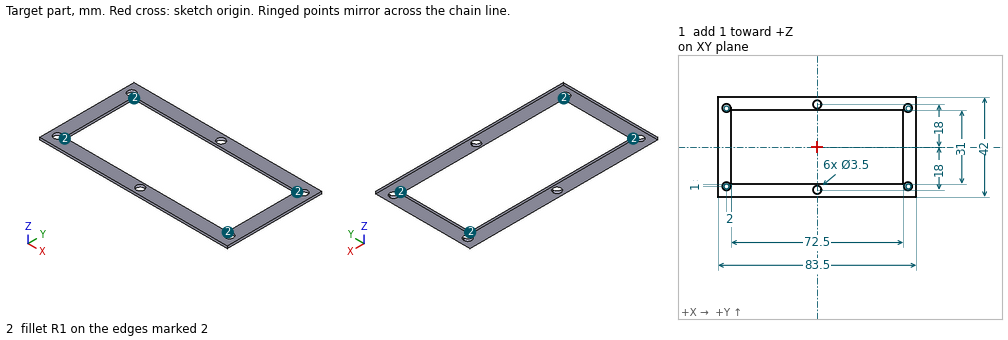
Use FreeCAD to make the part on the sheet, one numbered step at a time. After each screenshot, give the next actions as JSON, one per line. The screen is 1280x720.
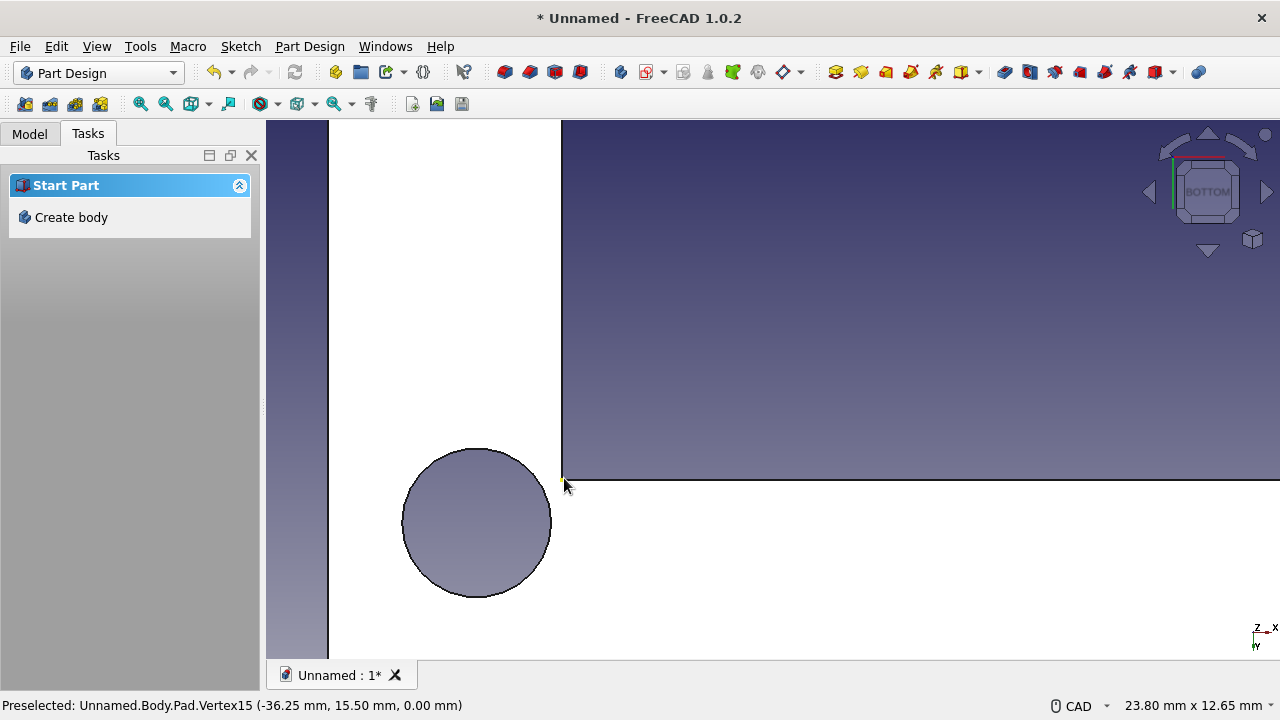
{"action": "left_click", "coordinate": [141, 104]}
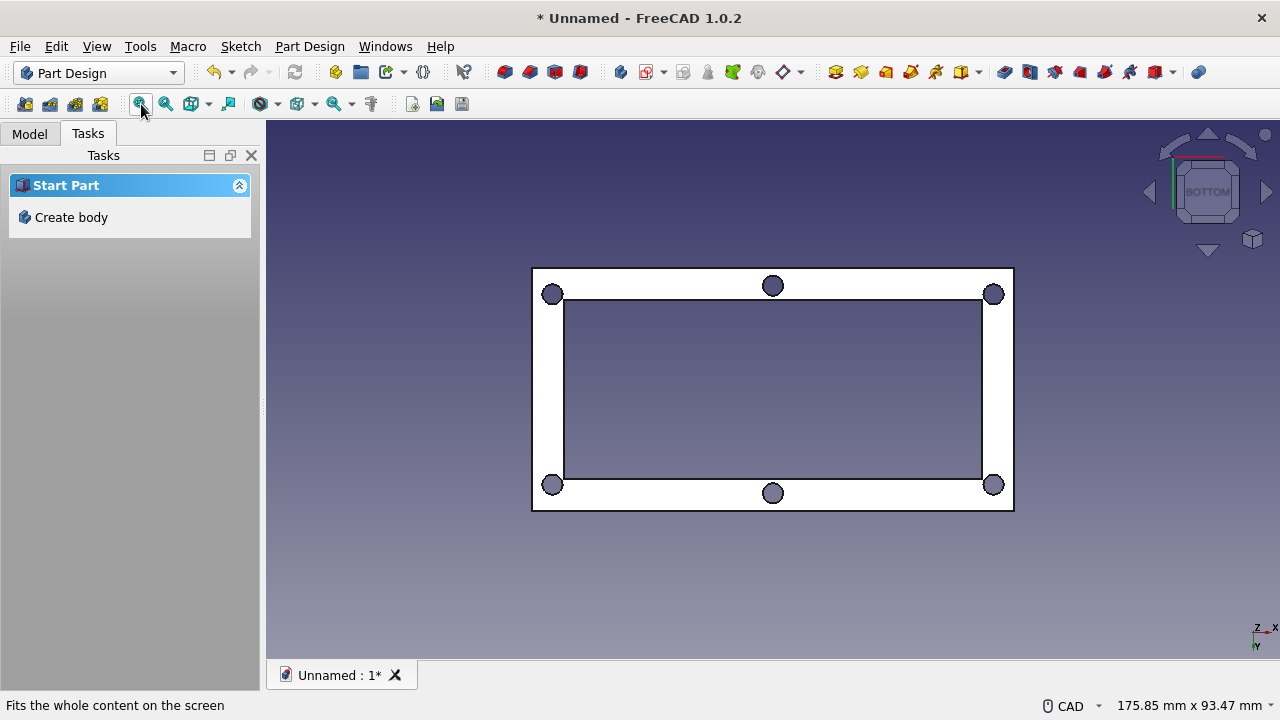
{"action": "key", "text": "4"}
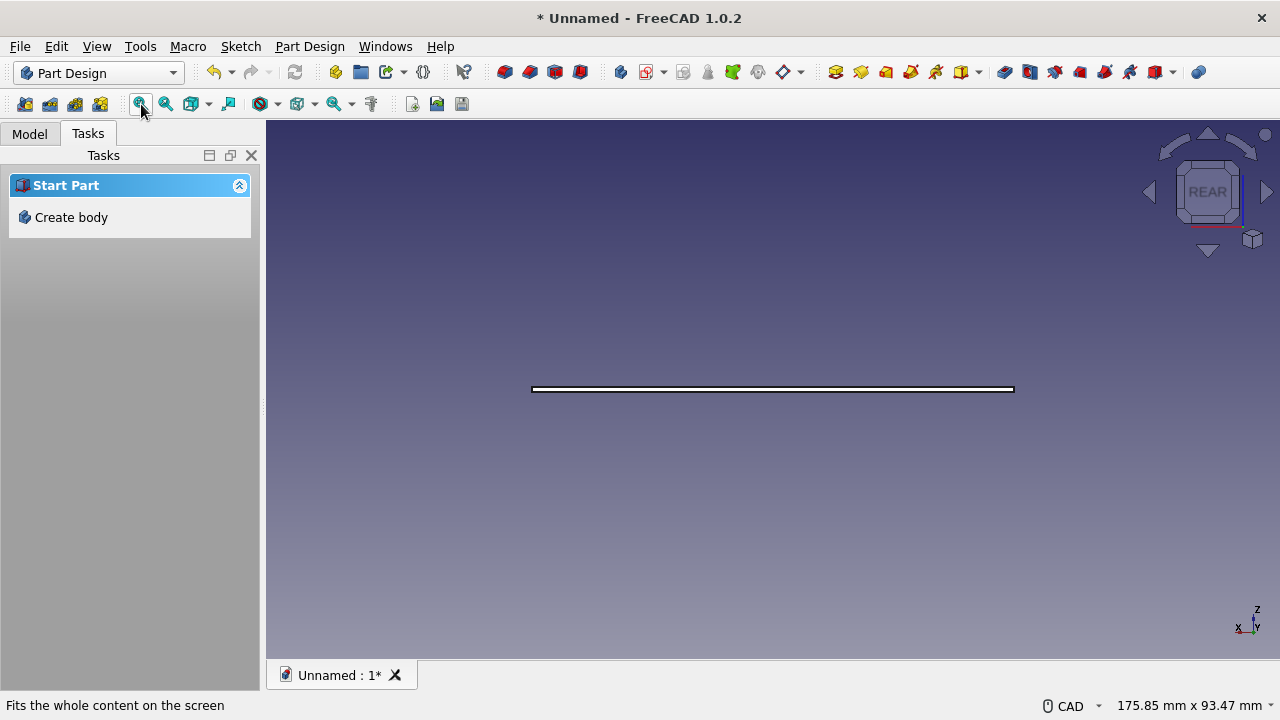
{"action": "scroll", "coordinate": [982, 389], "scroll_direction": "up", "scroll_amount": 10}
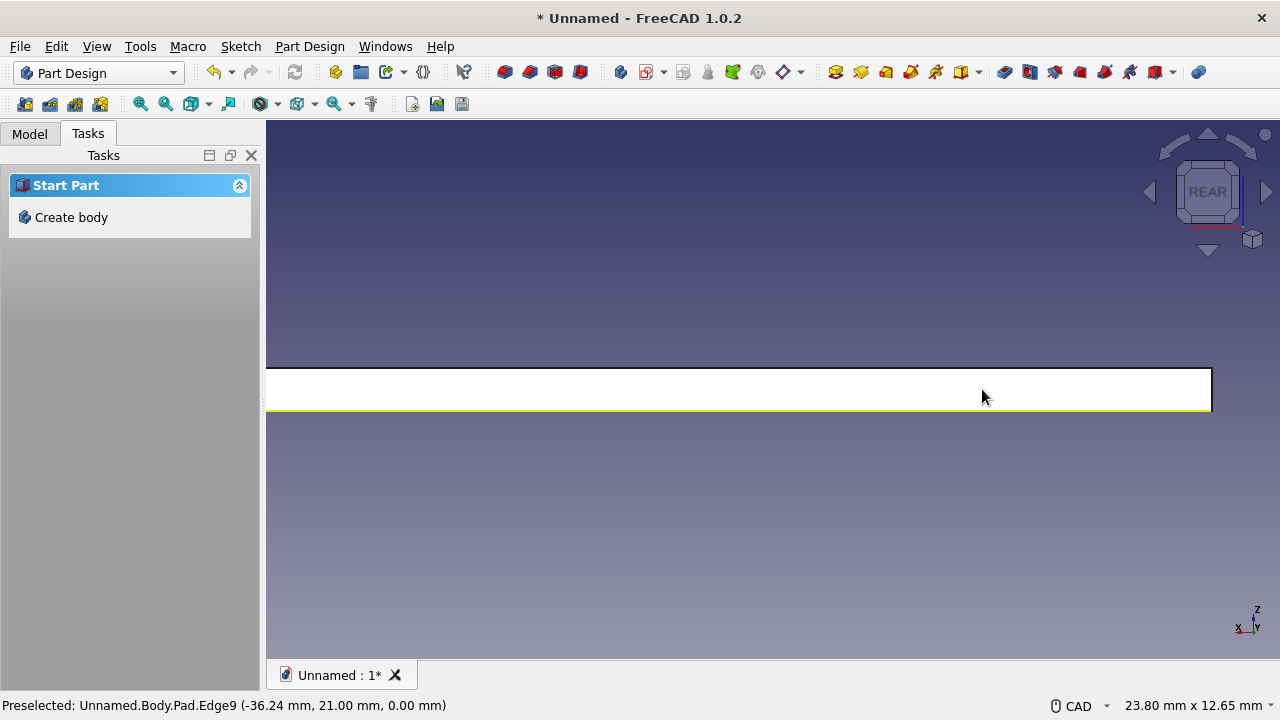
{"action": "key", "text": "v f"}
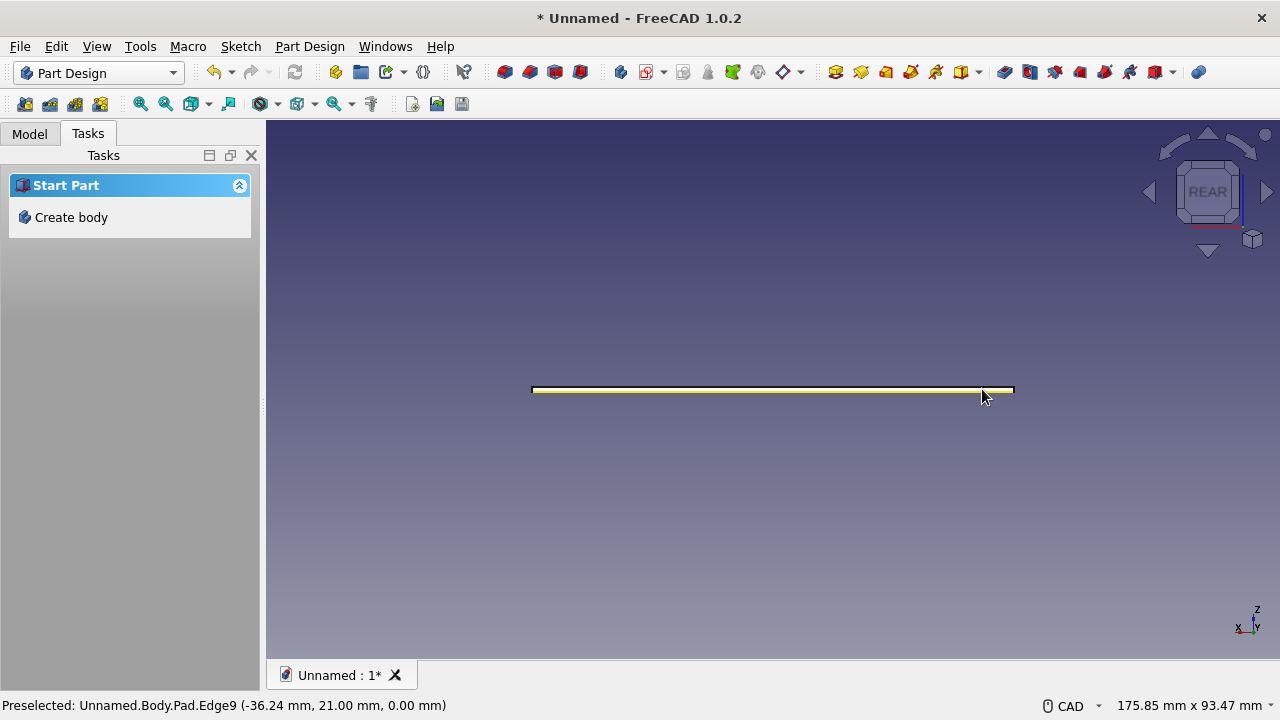
{"action": "key", "text": "6"}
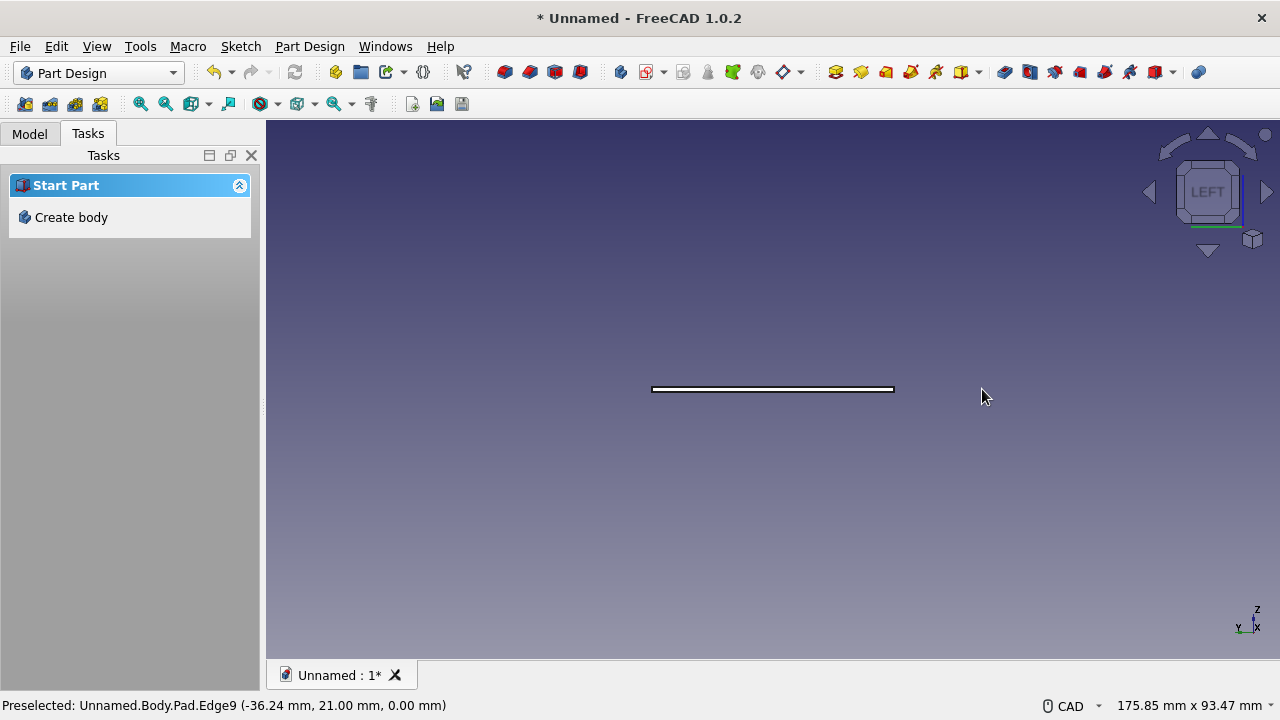
{"action": "left_click", "coordinate": [141, 104]}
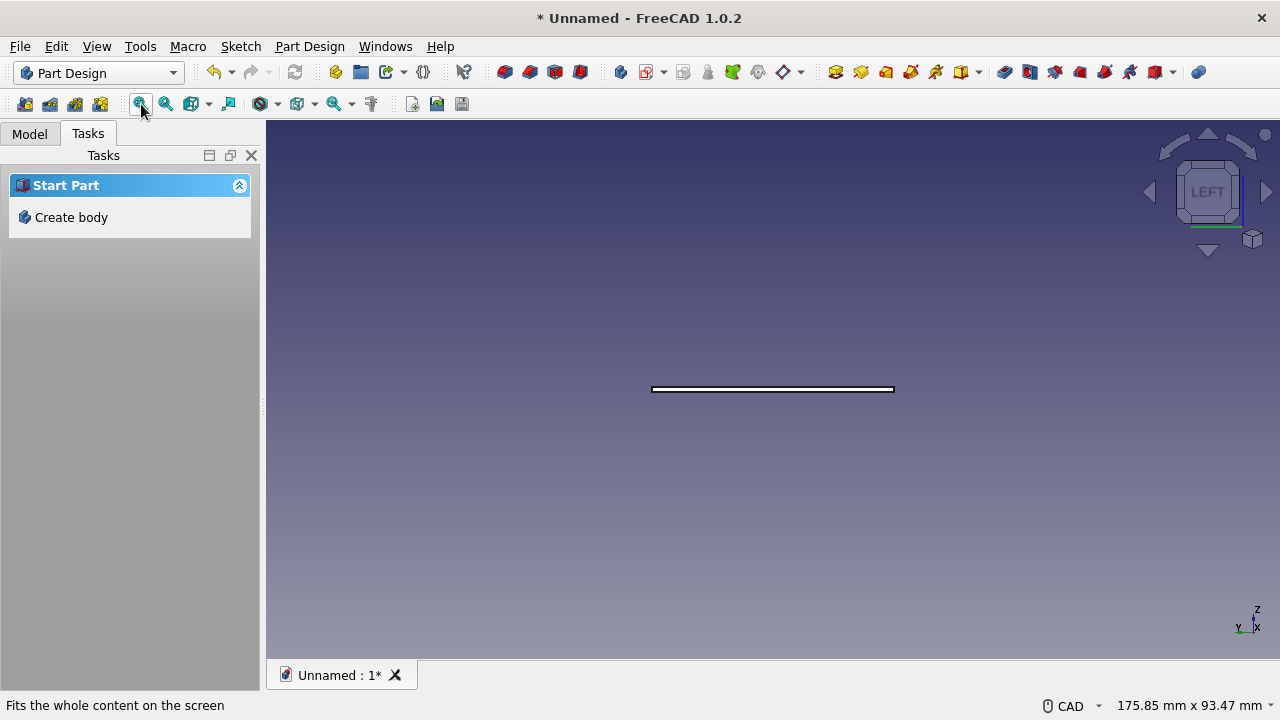
{"action": "scroll", "coordinate": [684, 388], "scroll_direction": "up", "scroll_amount": 10}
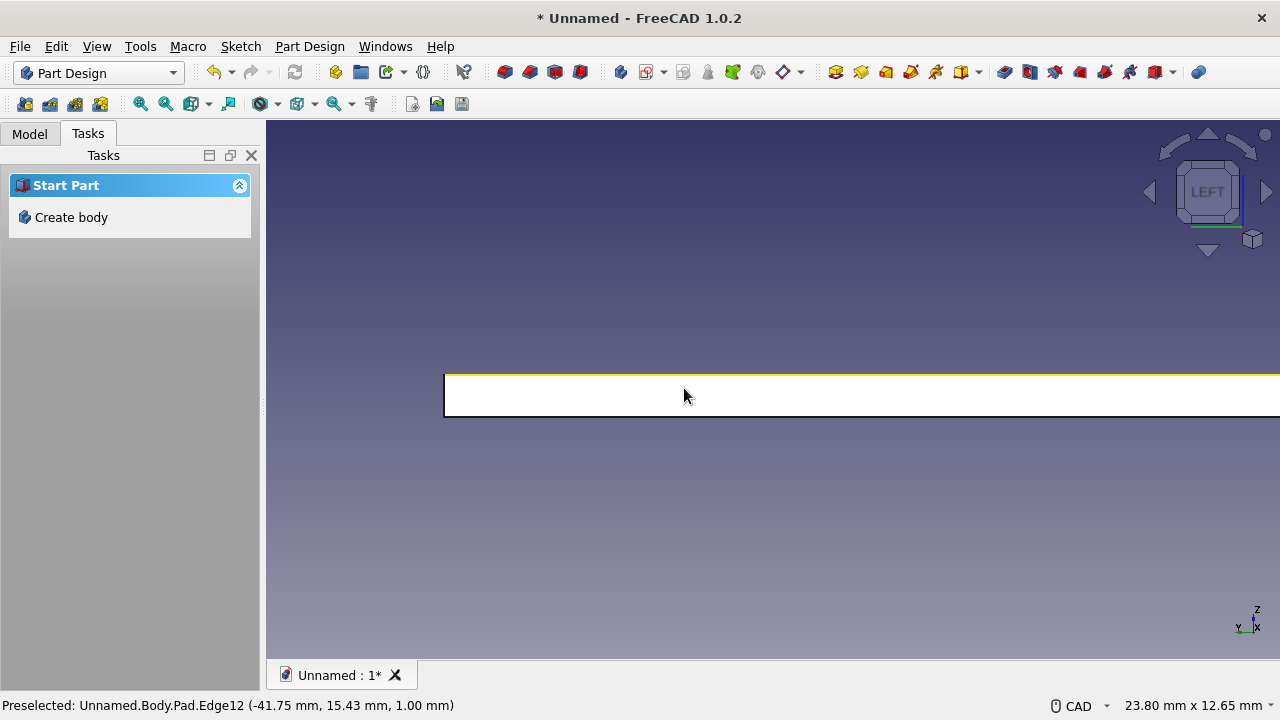
{"action": "key", "text": "v f"}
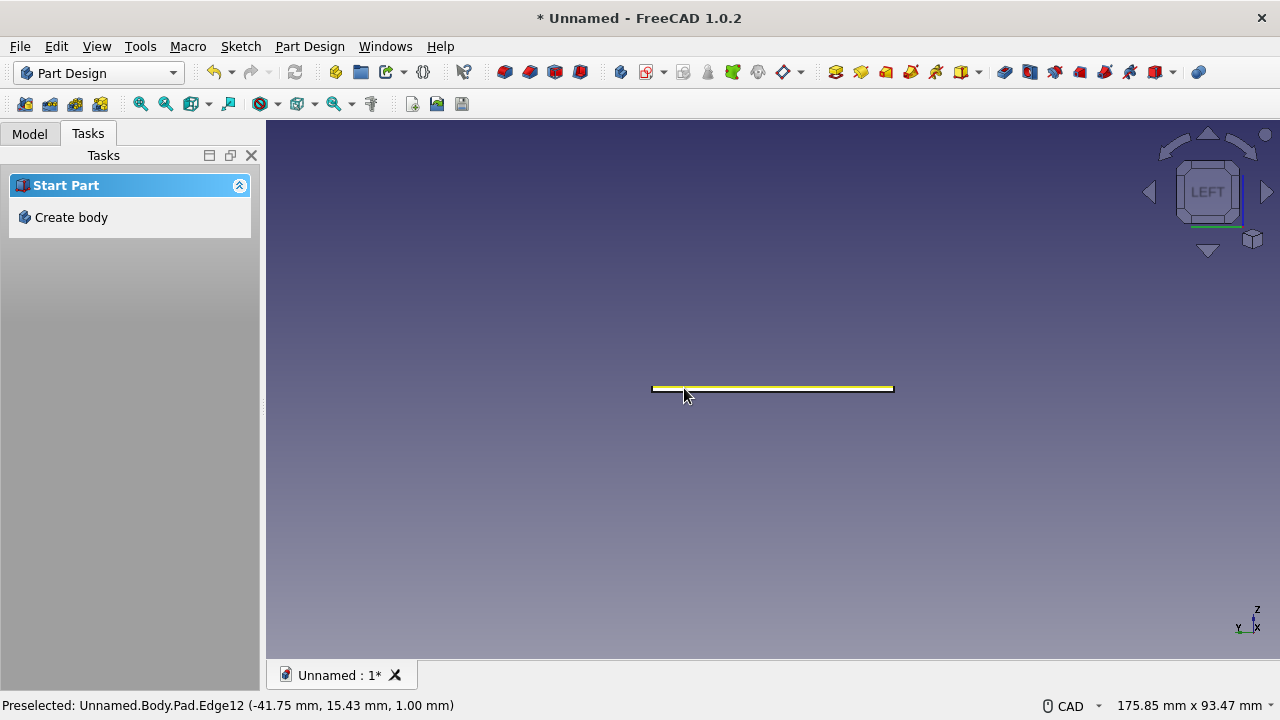
{"action": "key", "text": "v 3"}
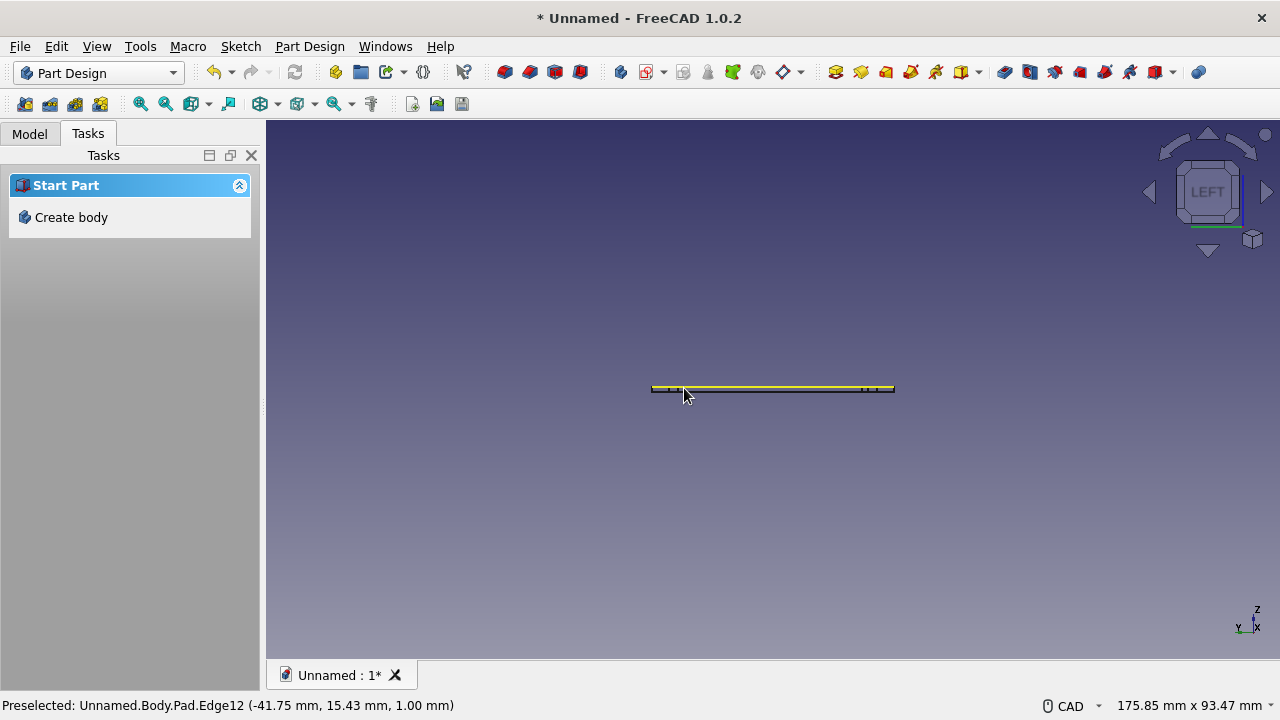
{"action": "key", "text": "0"}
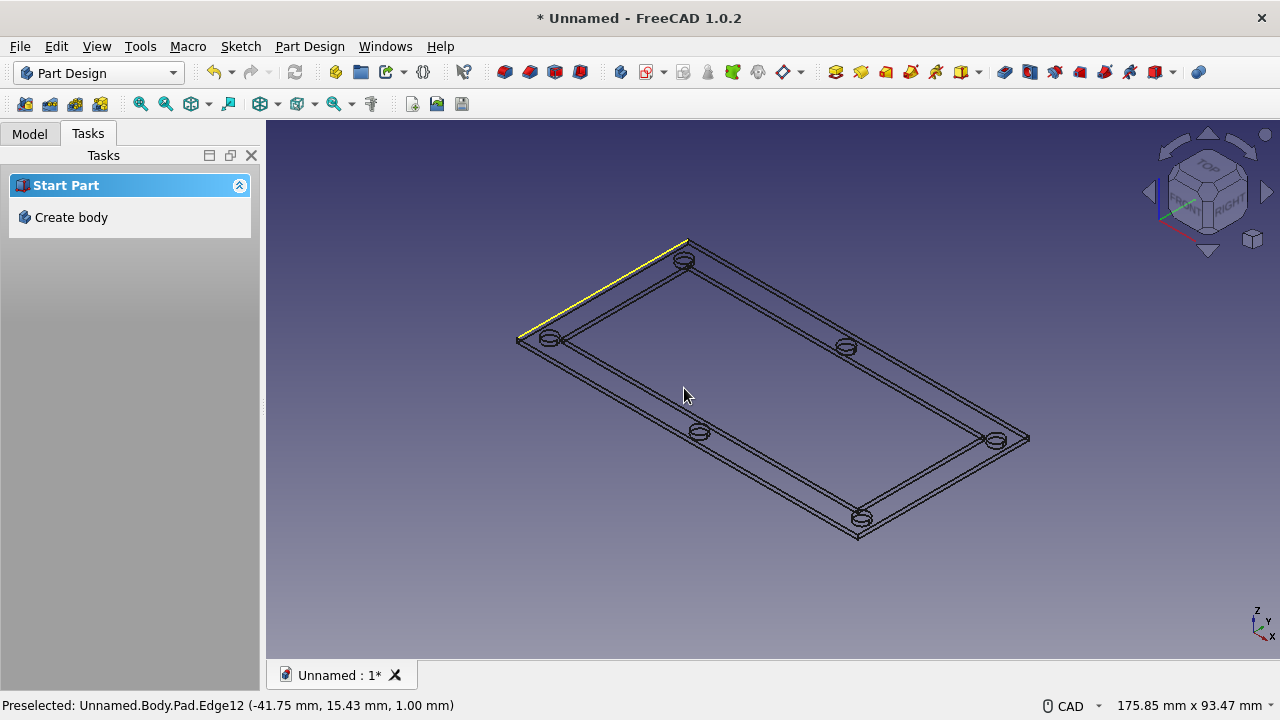
{"action": "scroll", "coordinate": [688, 267], "scroll_direction": "up", "scroll_amount": 10}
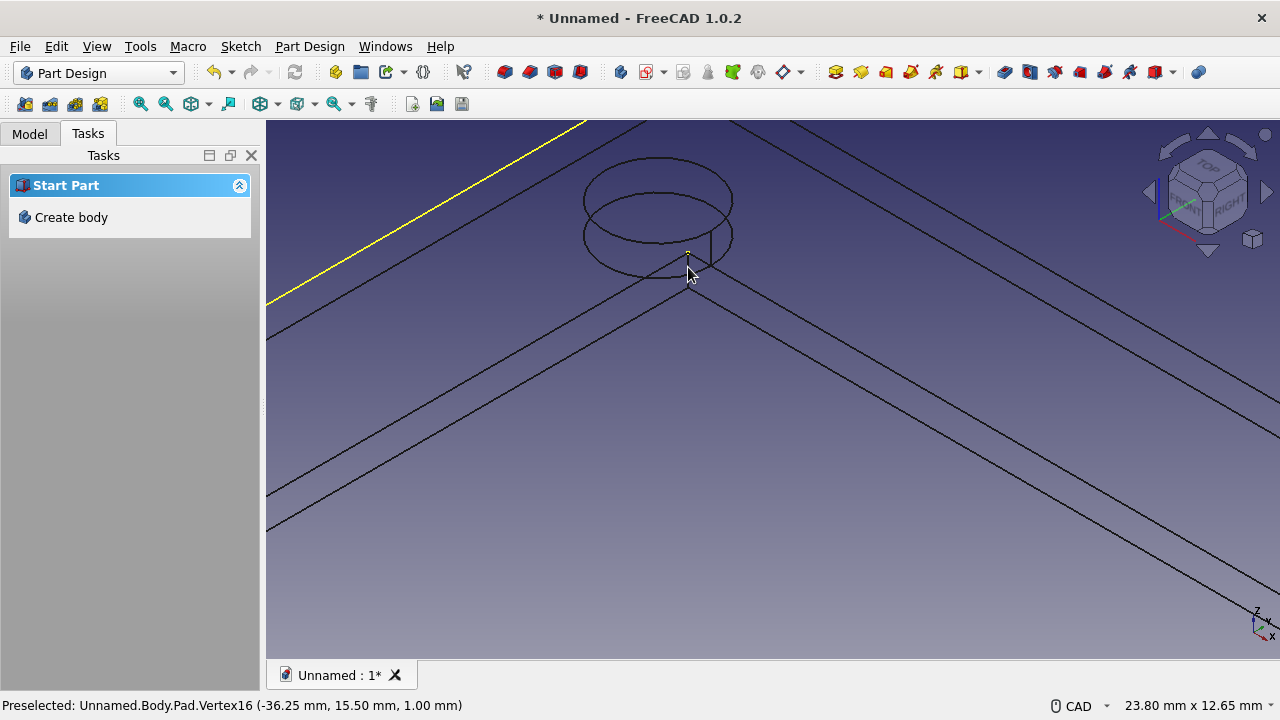
{"action": "left_click", "coordinate": [688, 269]}